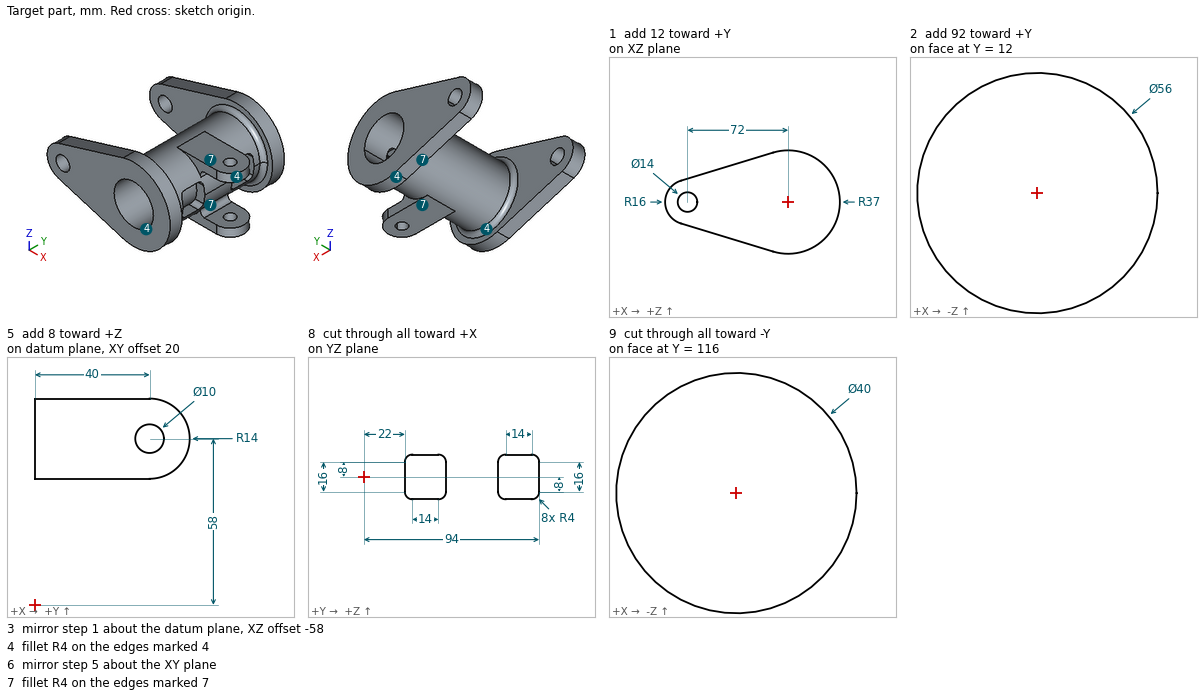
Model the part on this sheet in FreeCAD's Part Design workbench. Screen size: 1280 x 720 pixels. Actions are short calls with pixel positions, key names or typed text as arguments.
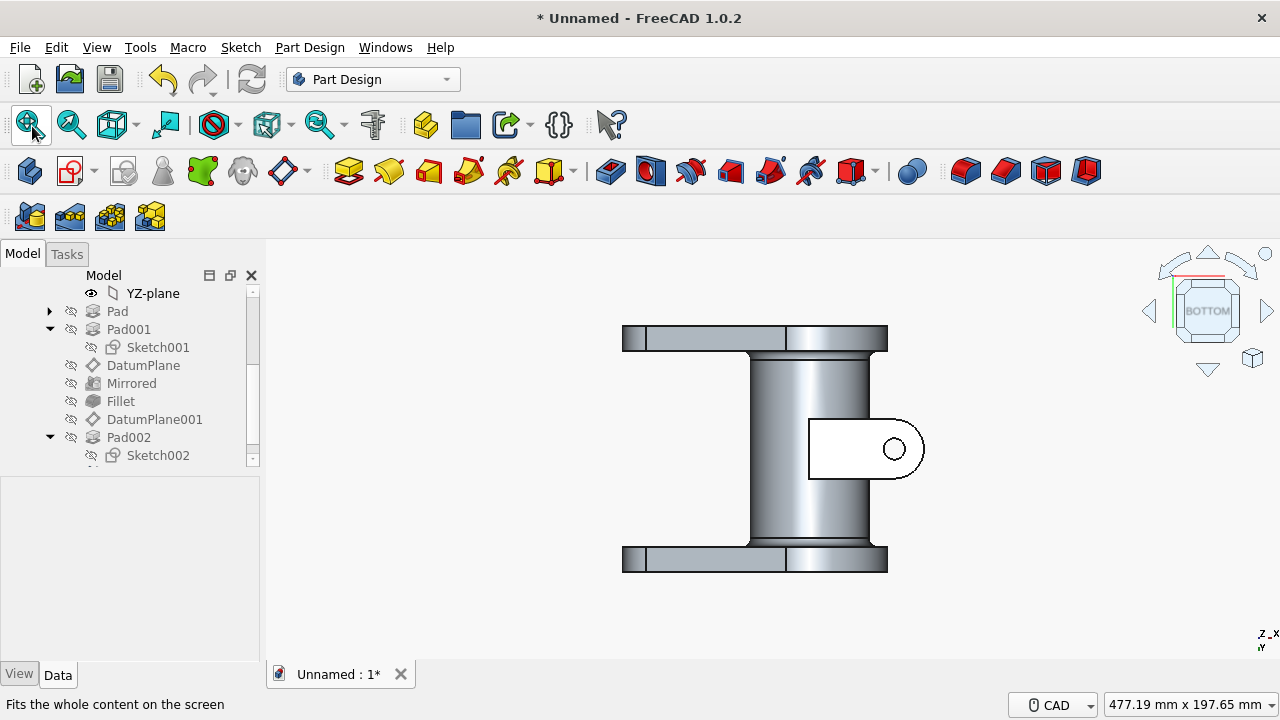
key(4)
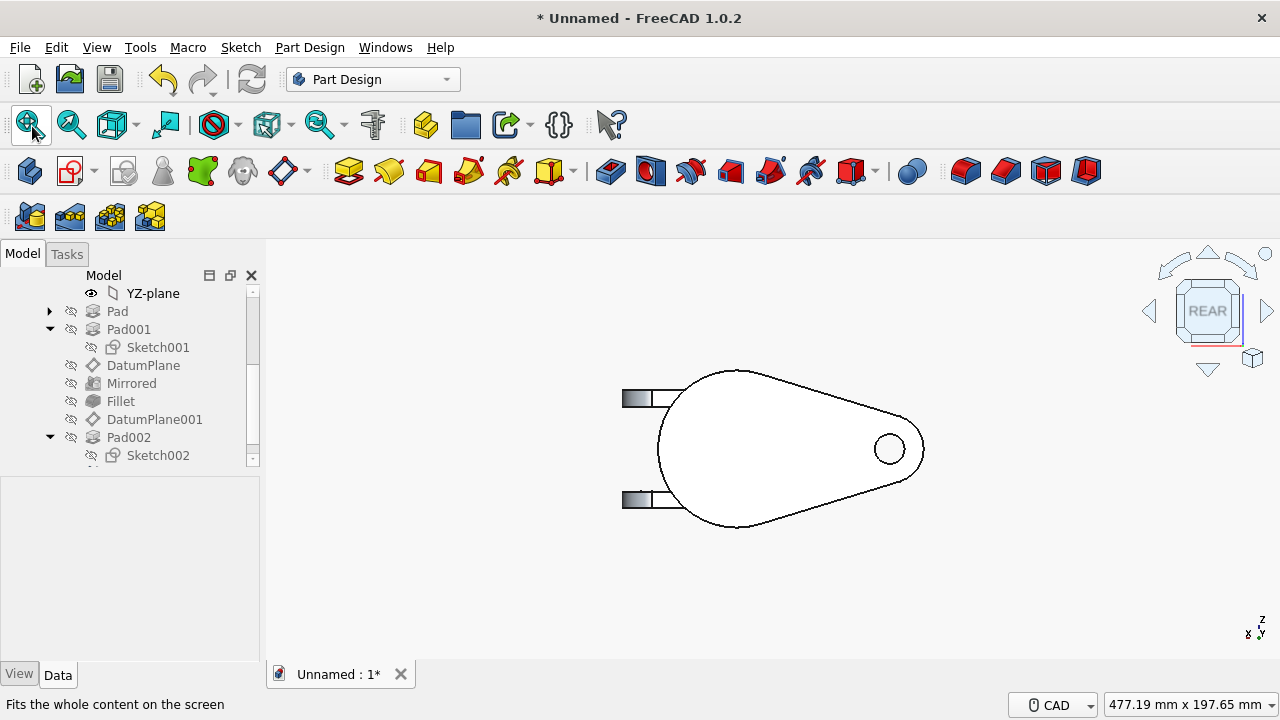
click(32, 126)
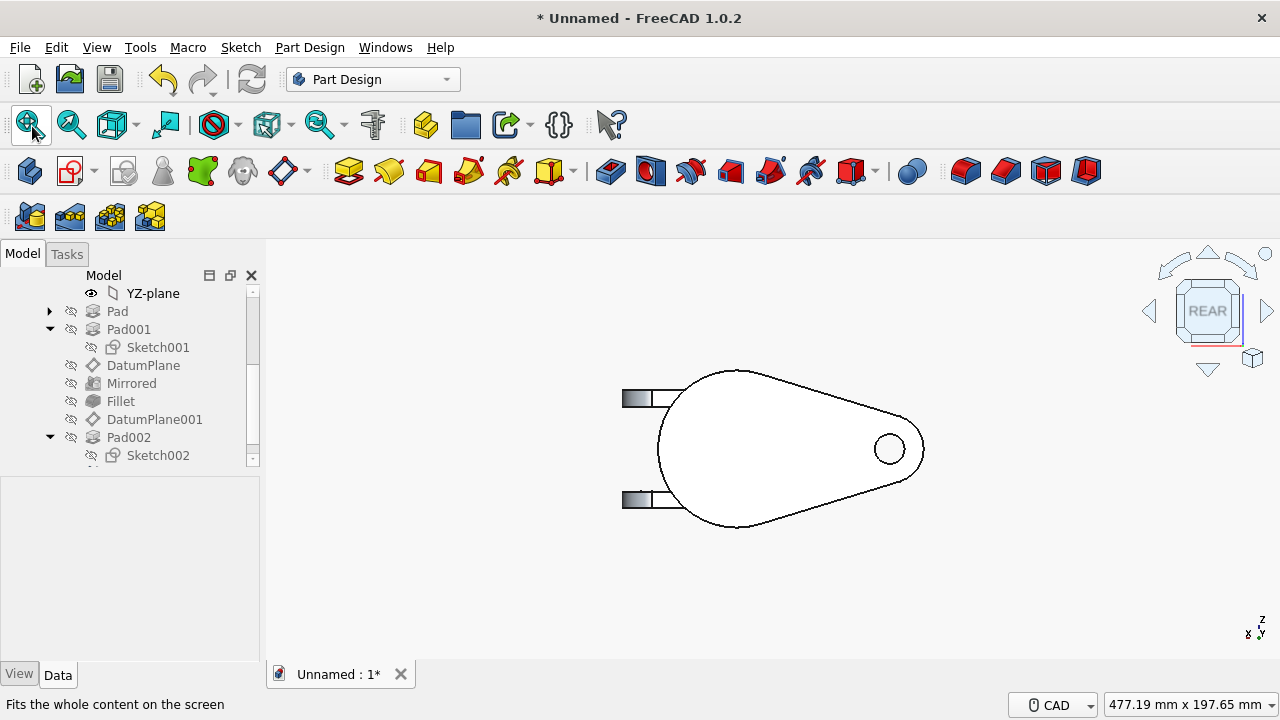
key(6)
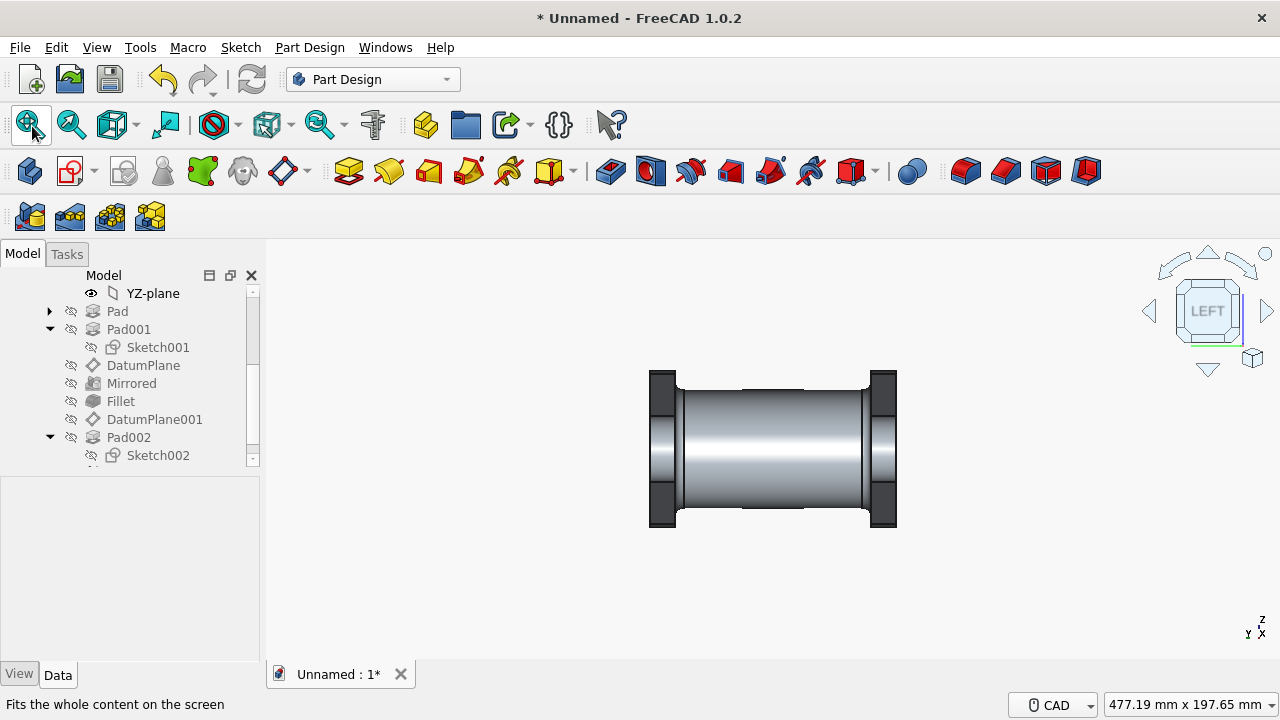
click(32, 126)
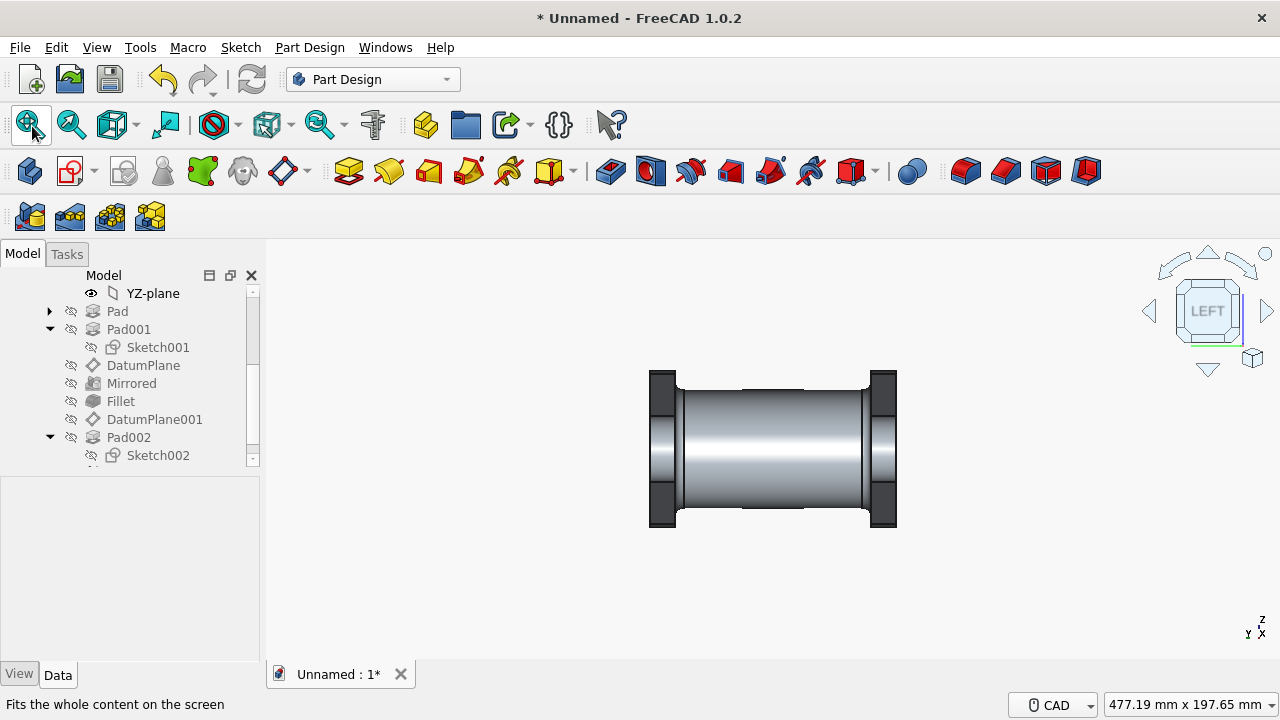
key(v)
key(3)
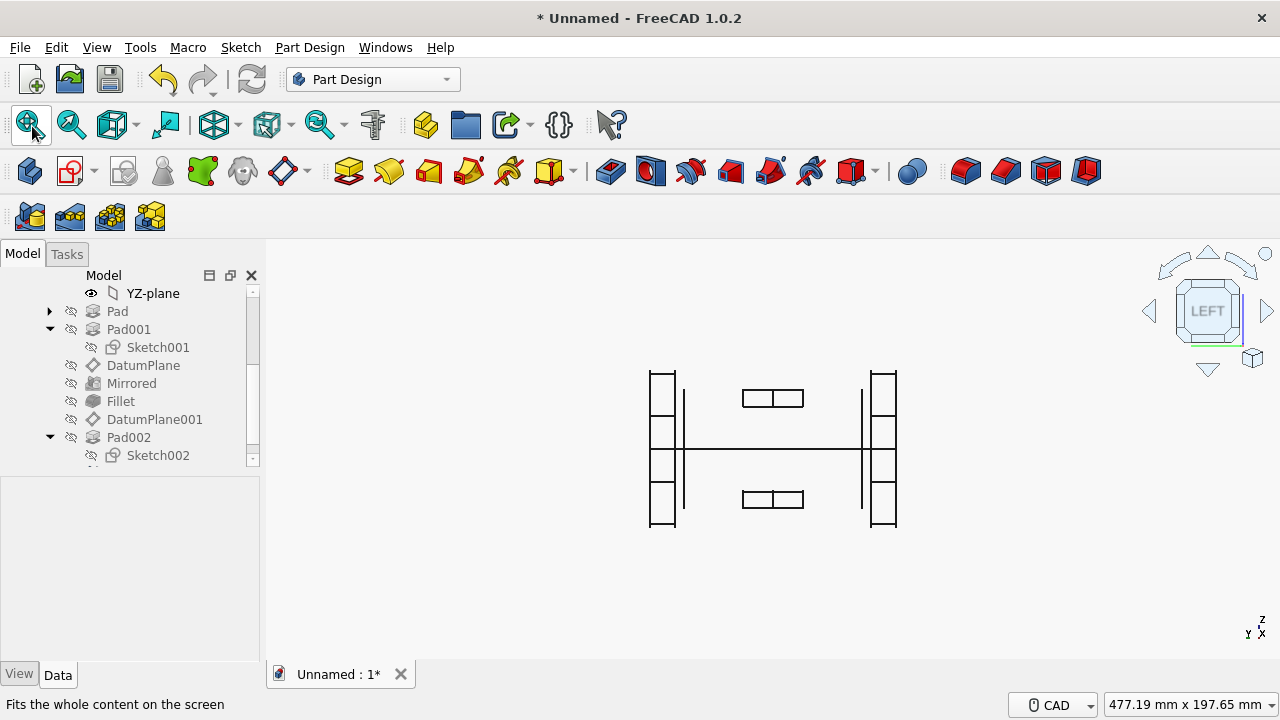
key(0)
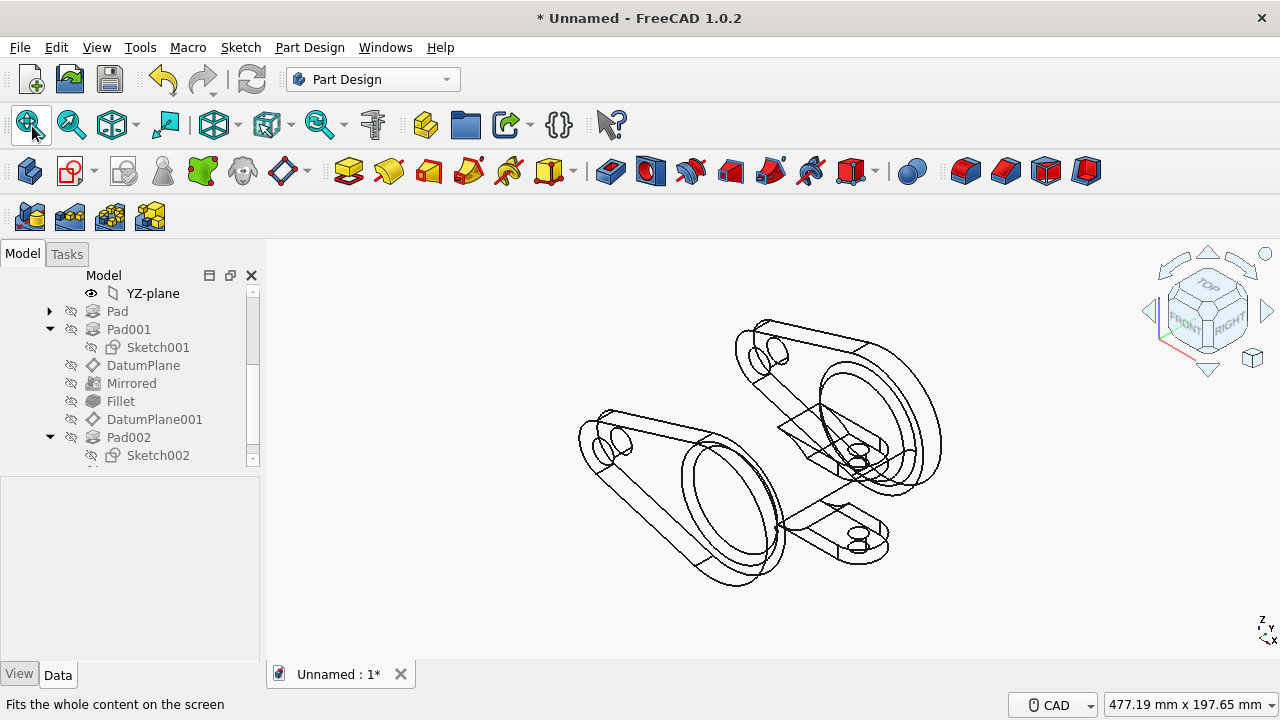
click(828, 445)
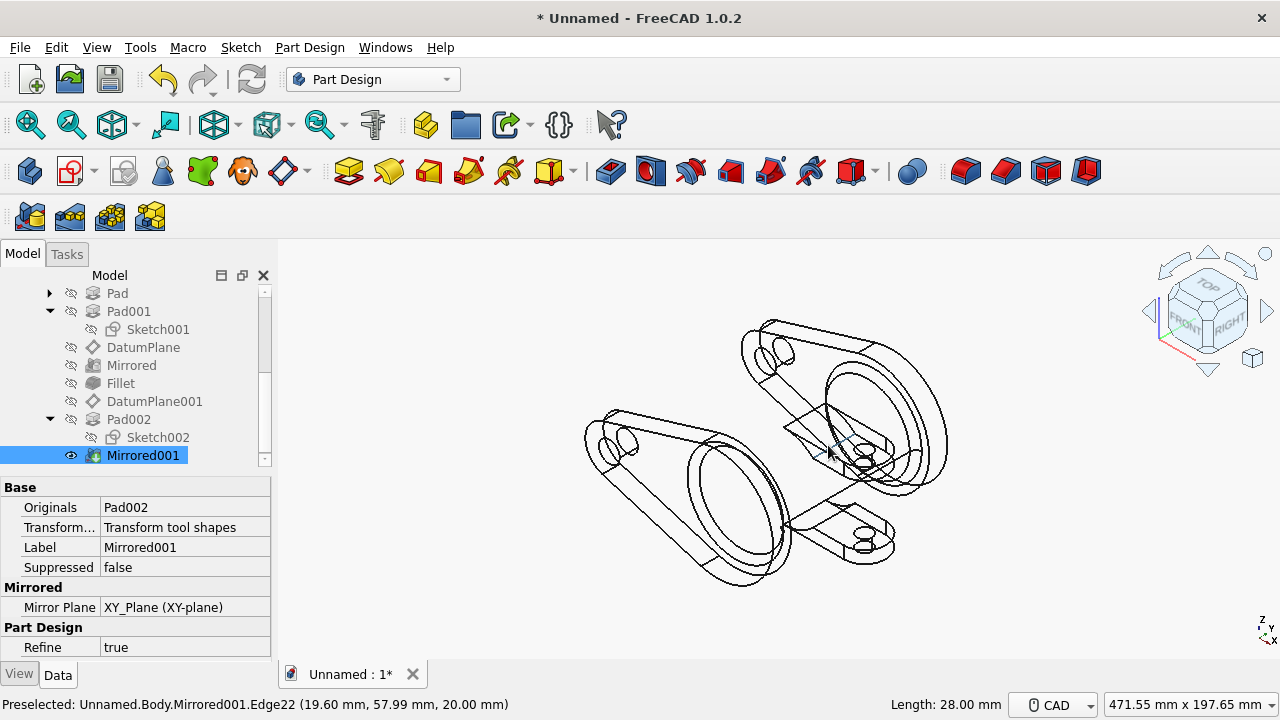
click(834, 514, ctrl)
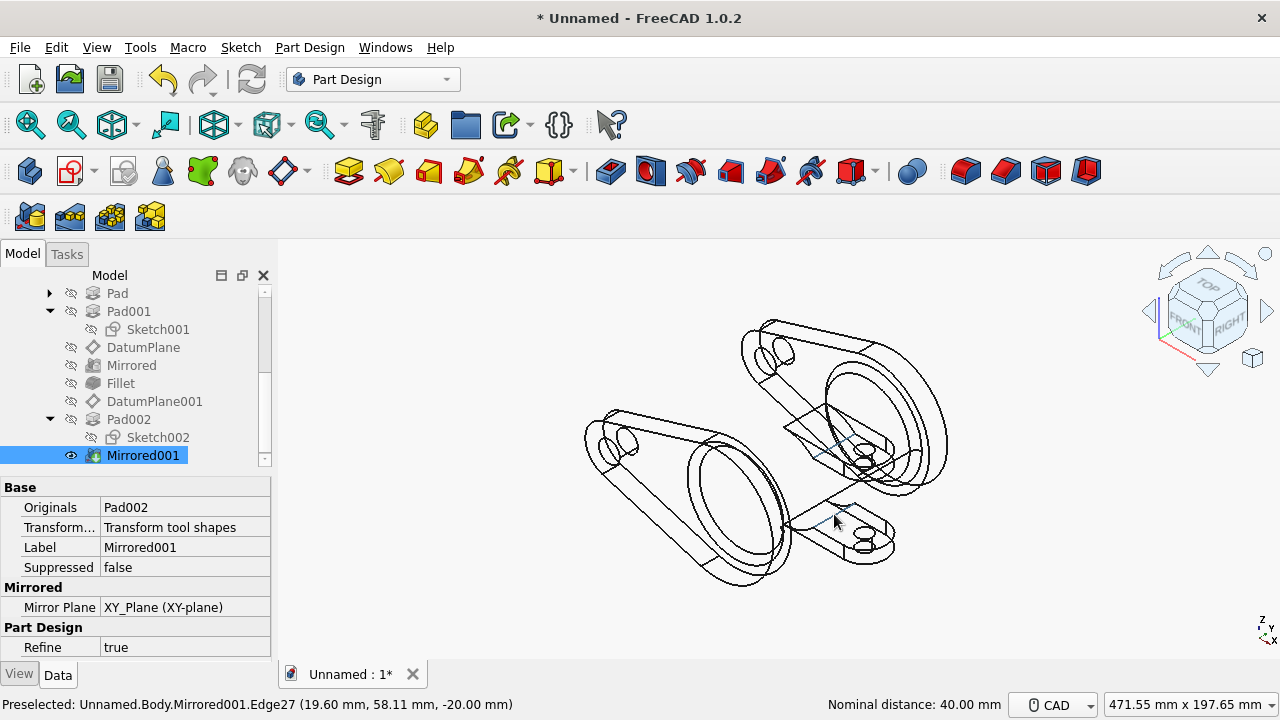
key(v)
key(1)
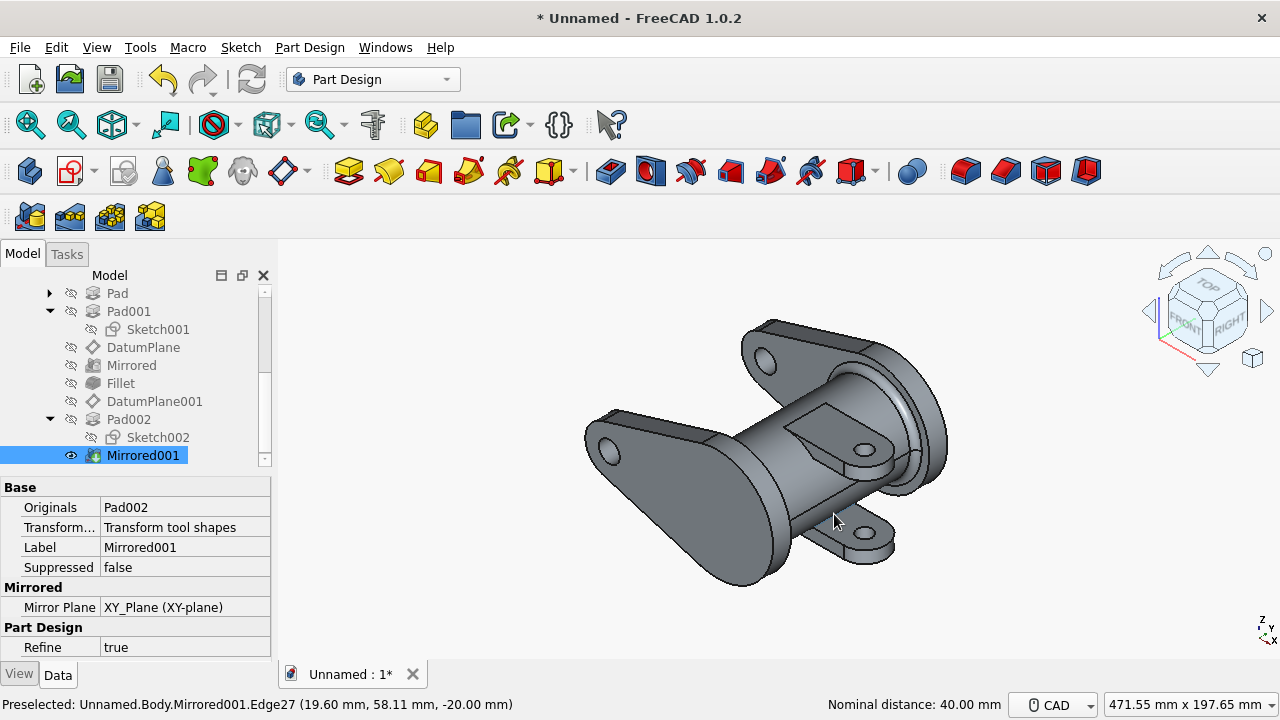
click(966, 172)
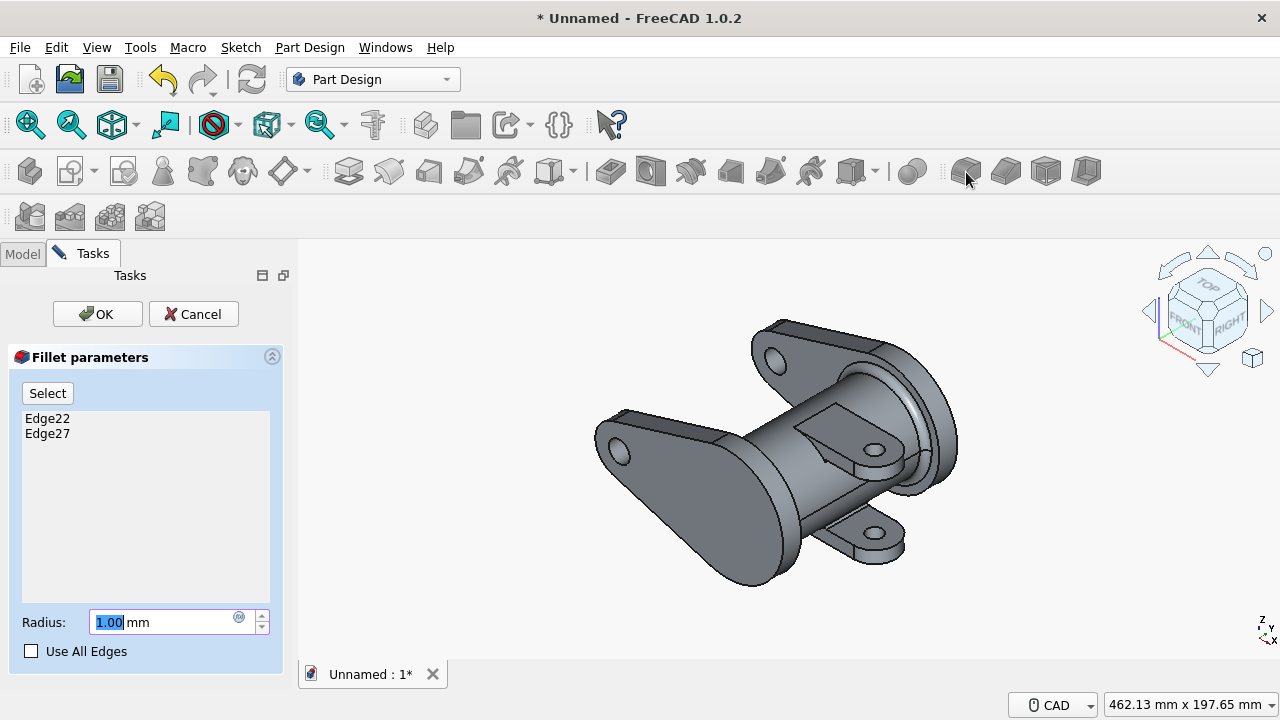
text(4)
key(Tab)